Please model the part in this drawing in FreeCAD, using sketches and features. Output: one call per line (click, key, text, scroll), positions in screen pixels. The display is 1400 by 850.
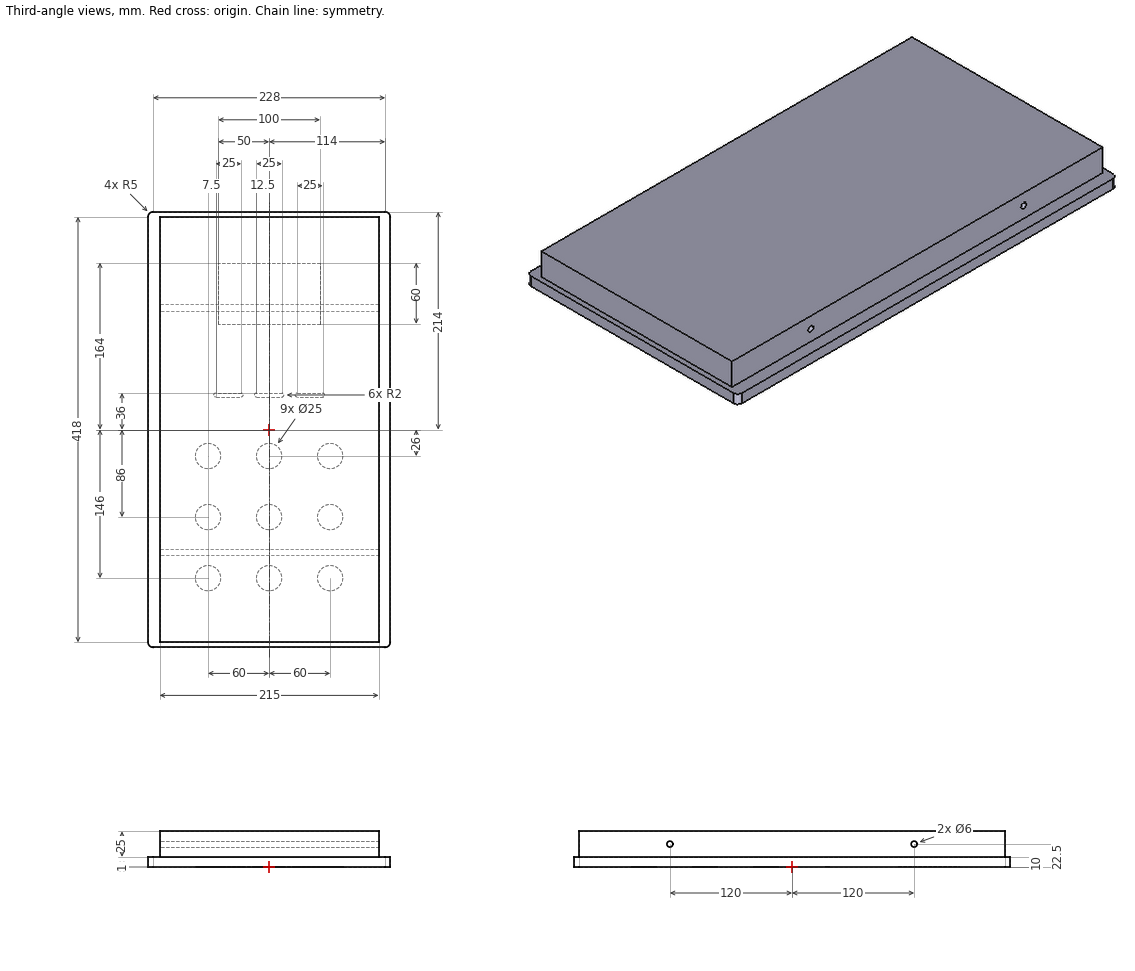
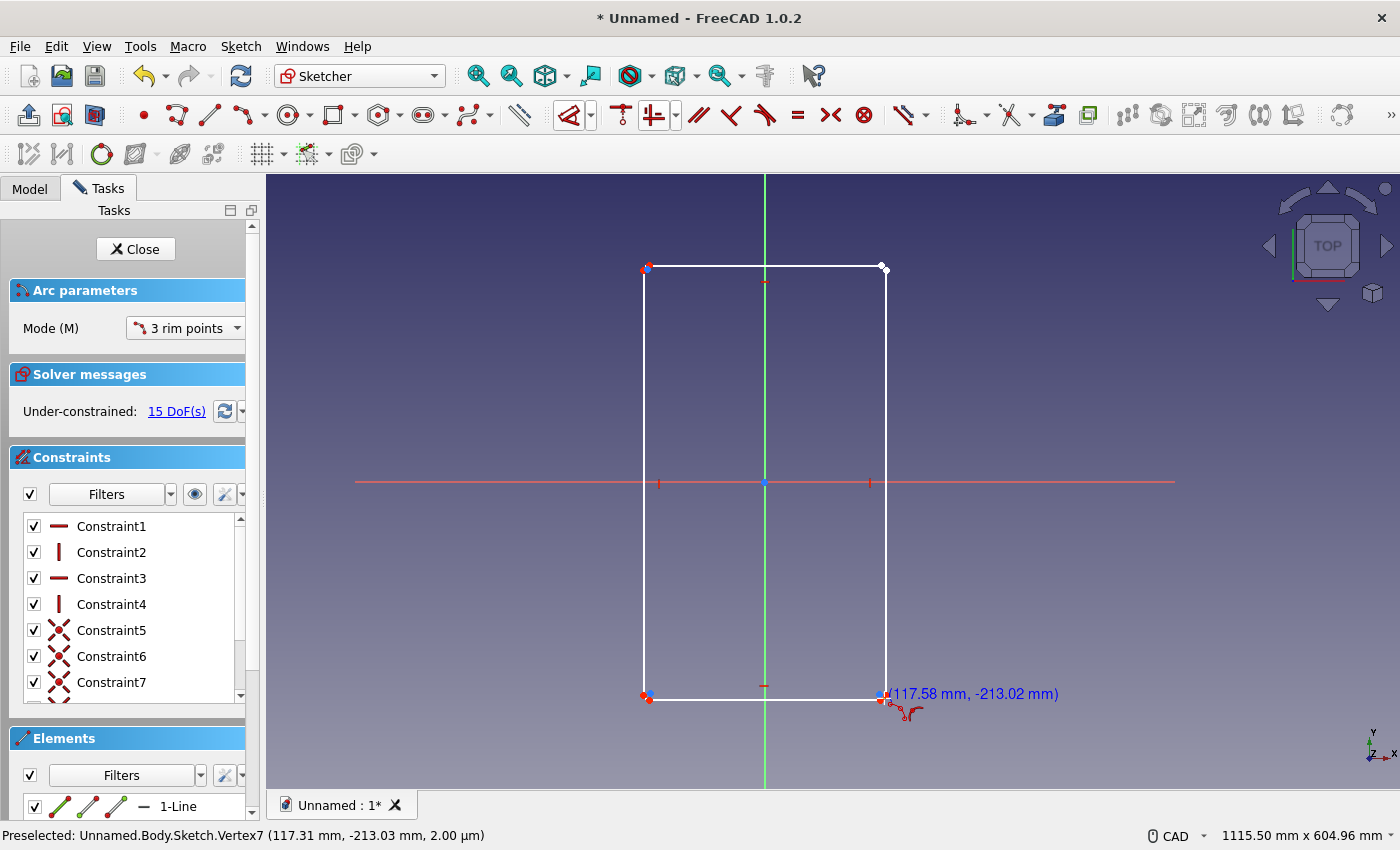
scroll(886, 270, up, 4)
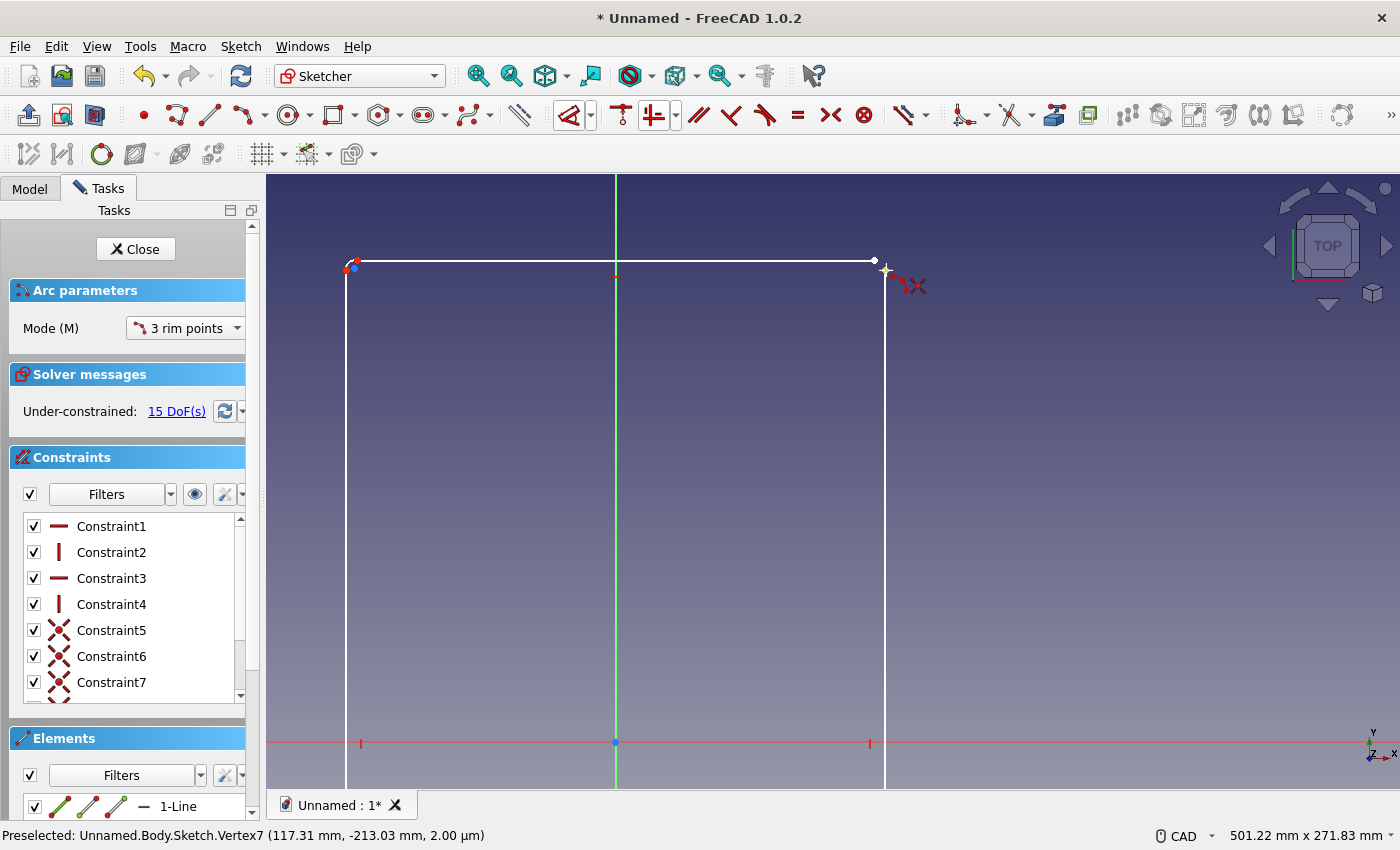
click(885, 271)
click(874, 261)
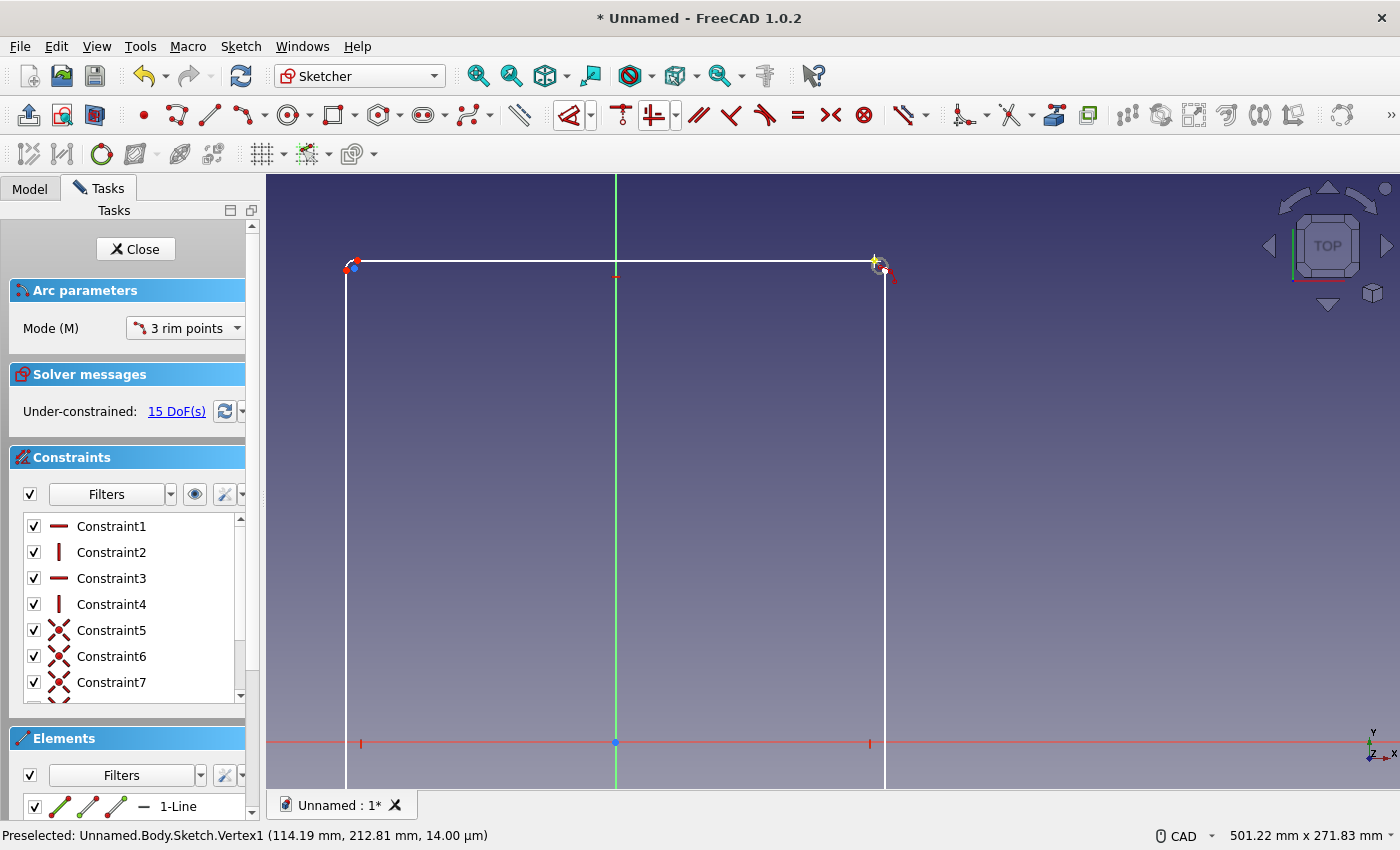
scroll(882, 261, up, 8)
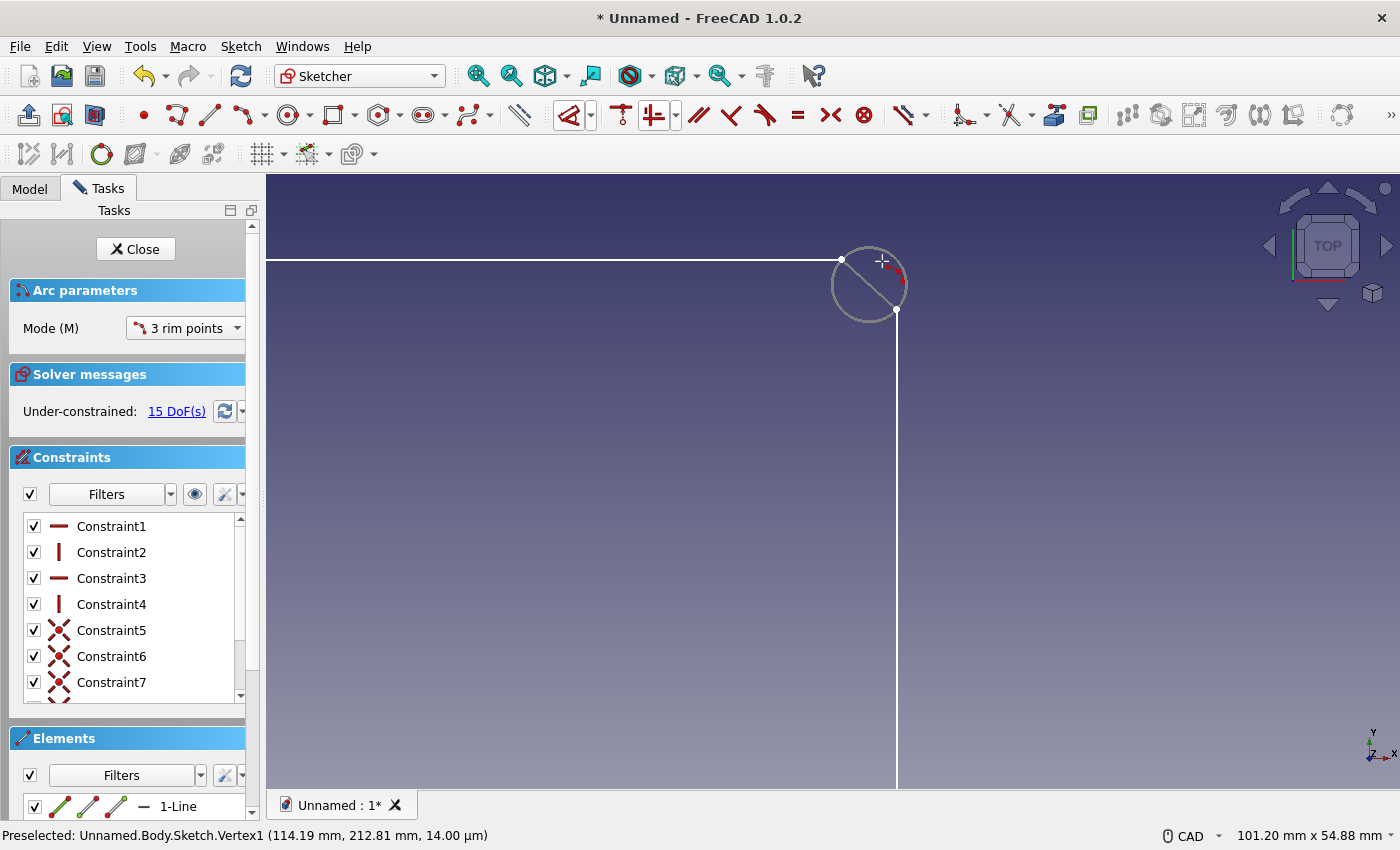
click(879, 263)
key(Escape)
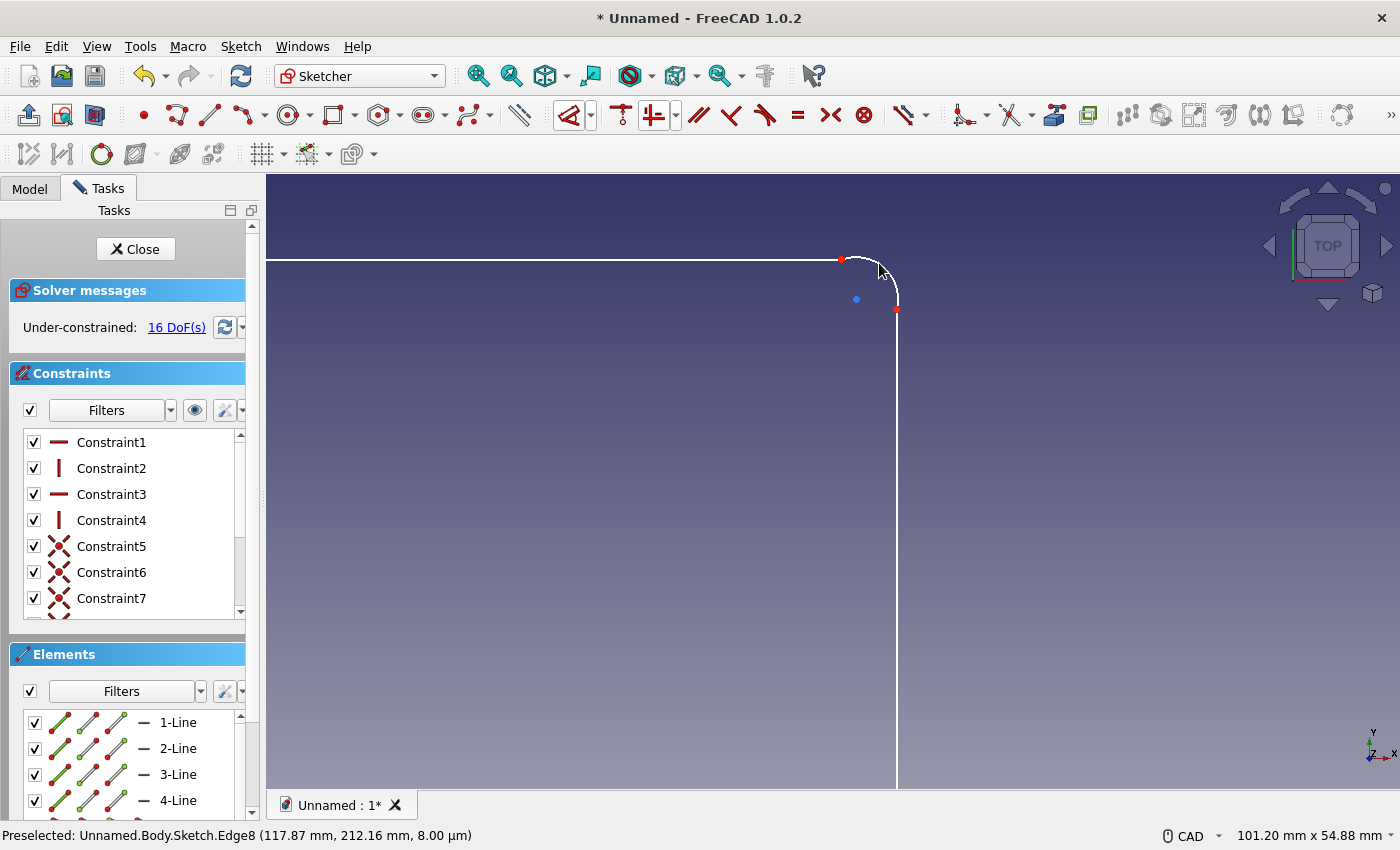
scroll(884, 266, down, 12)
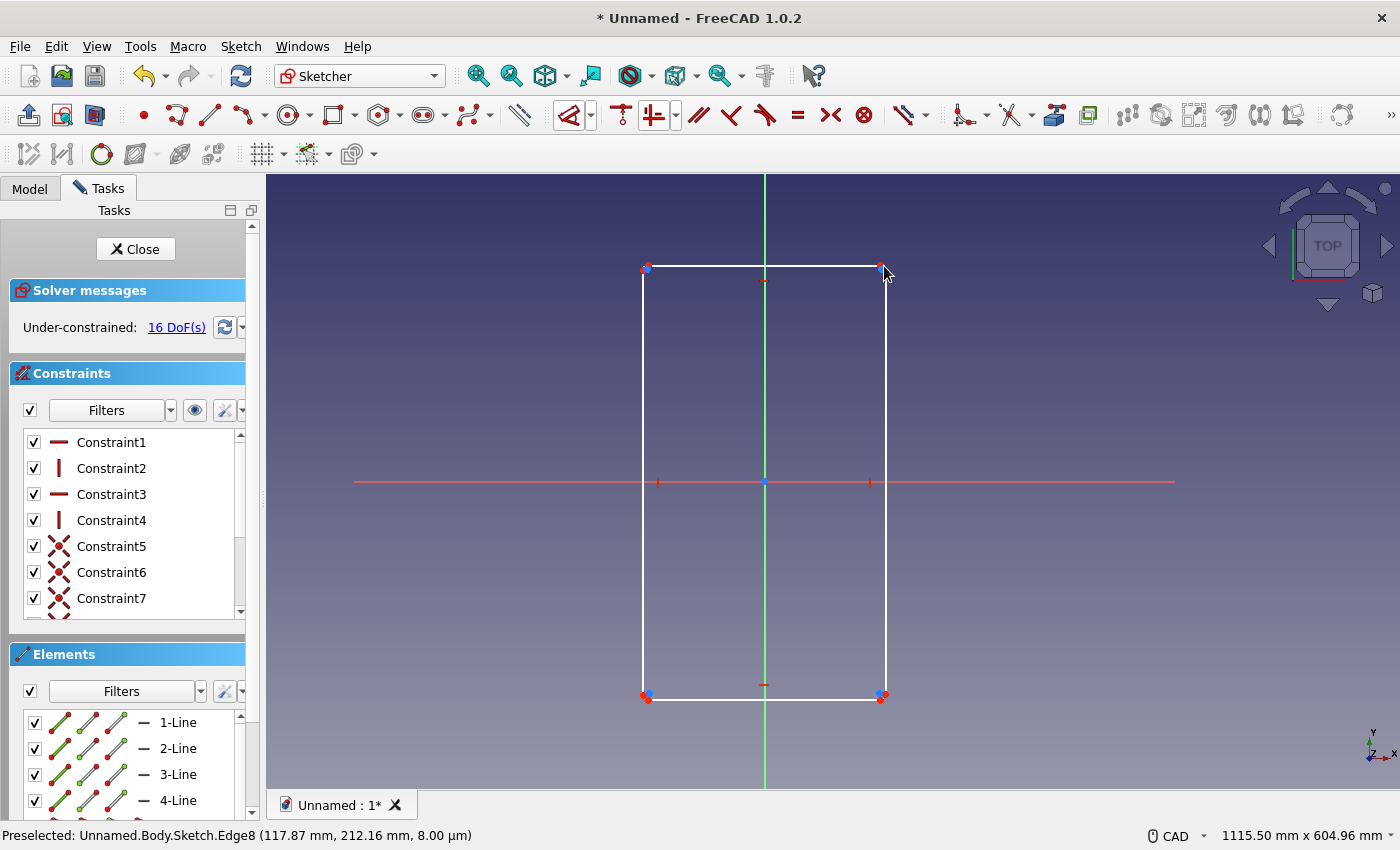
click(834, 266)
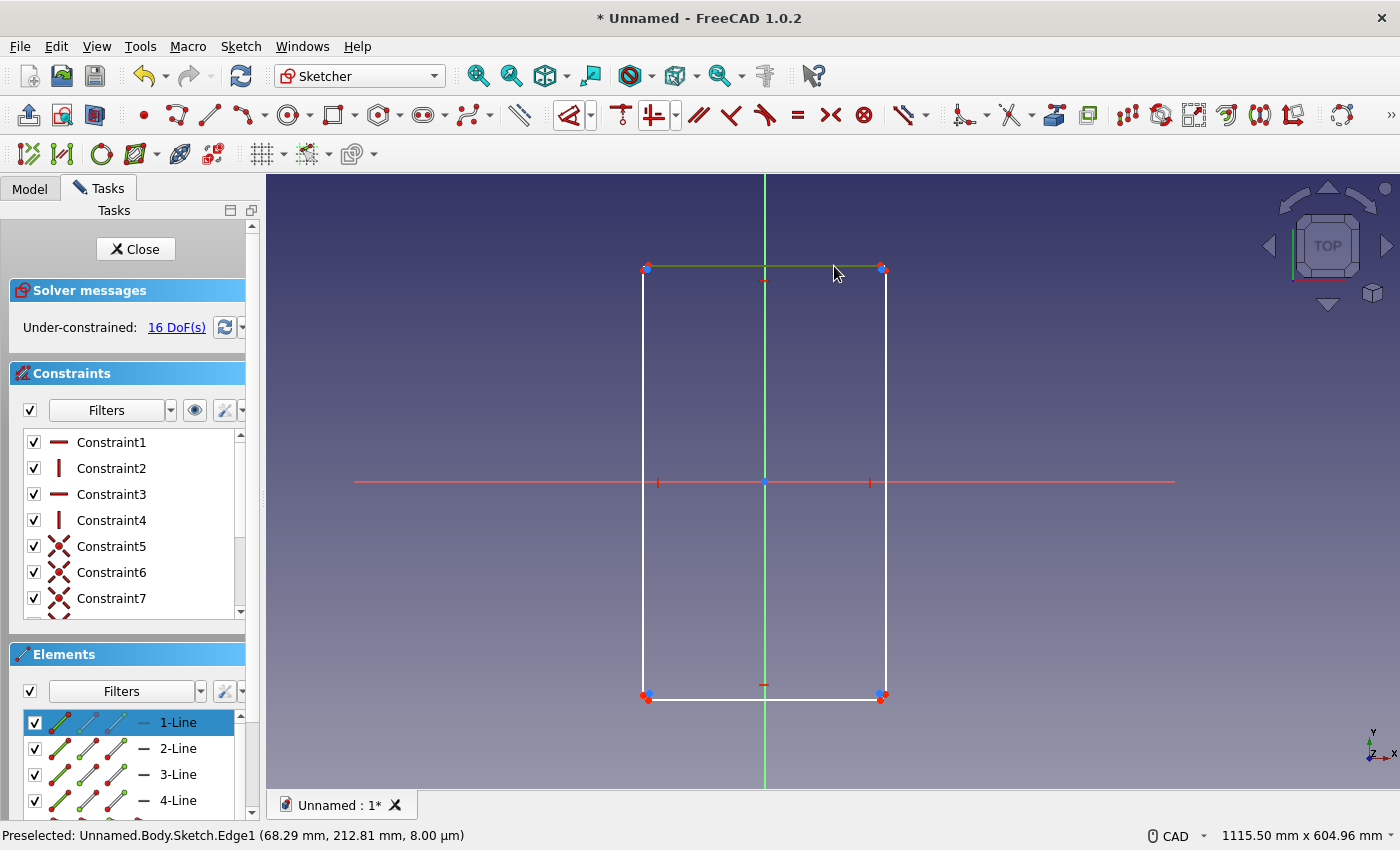
scroll(645, 266, up, 7)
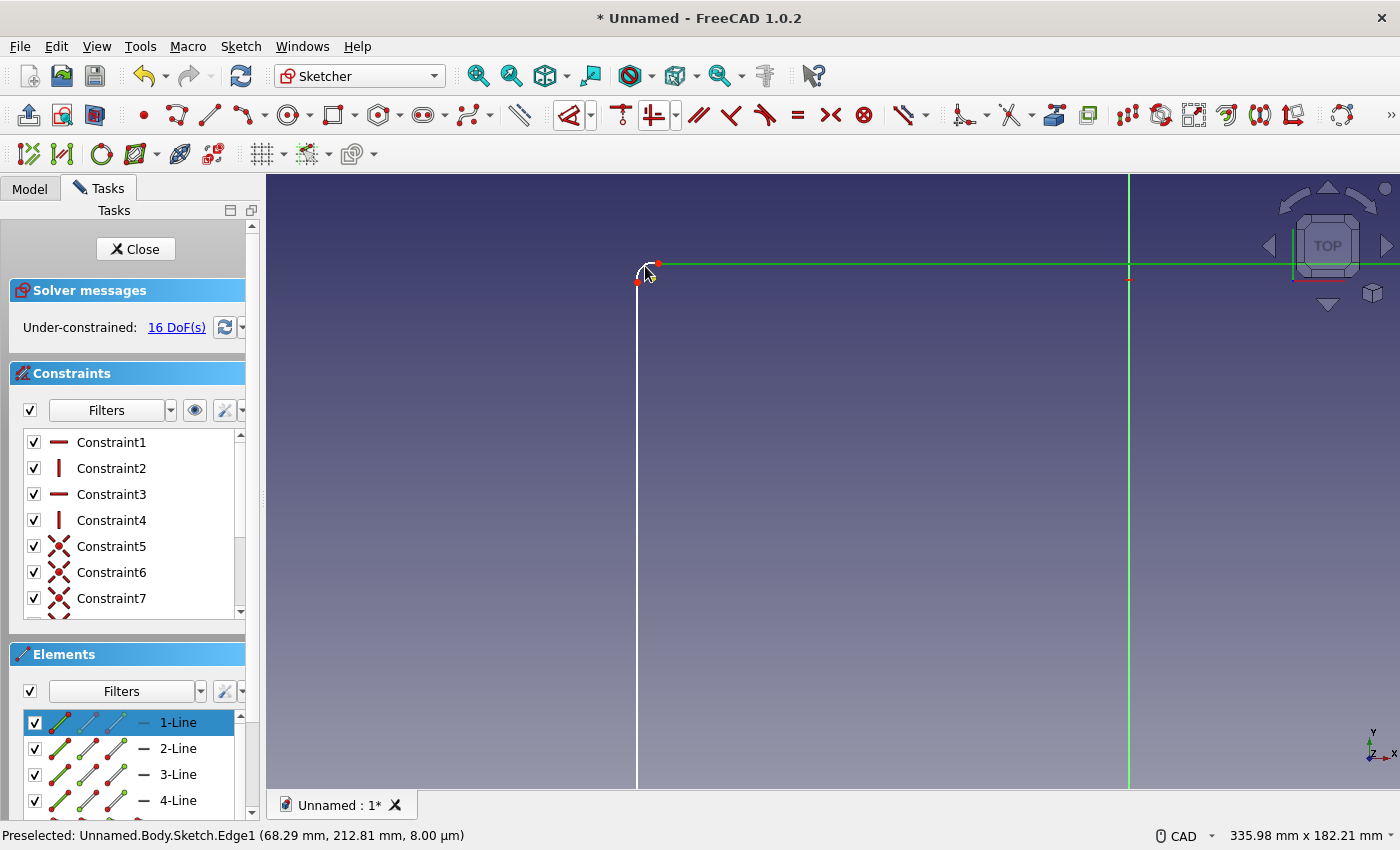
click(643, 266)